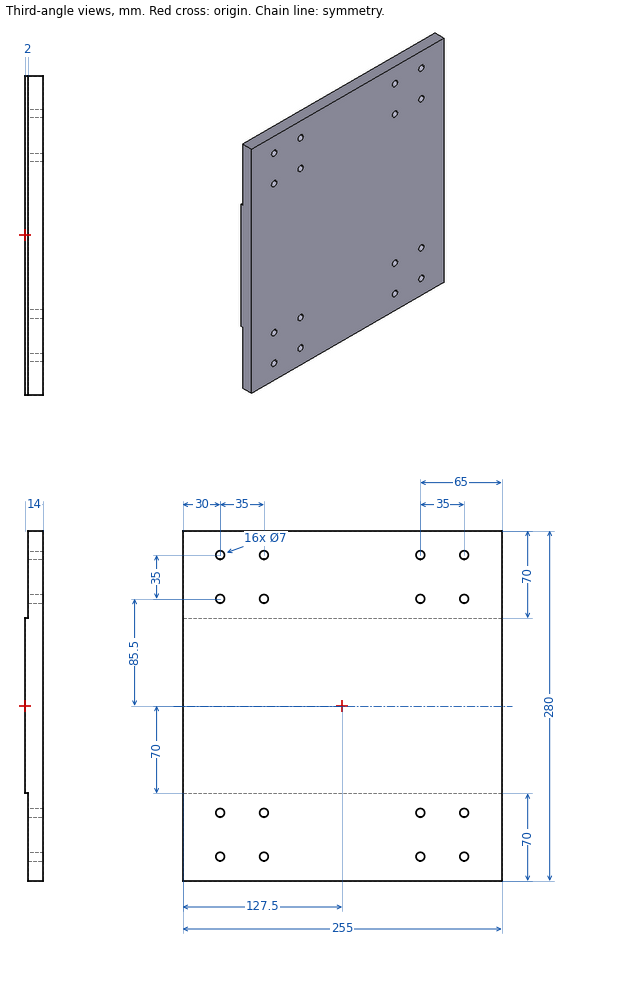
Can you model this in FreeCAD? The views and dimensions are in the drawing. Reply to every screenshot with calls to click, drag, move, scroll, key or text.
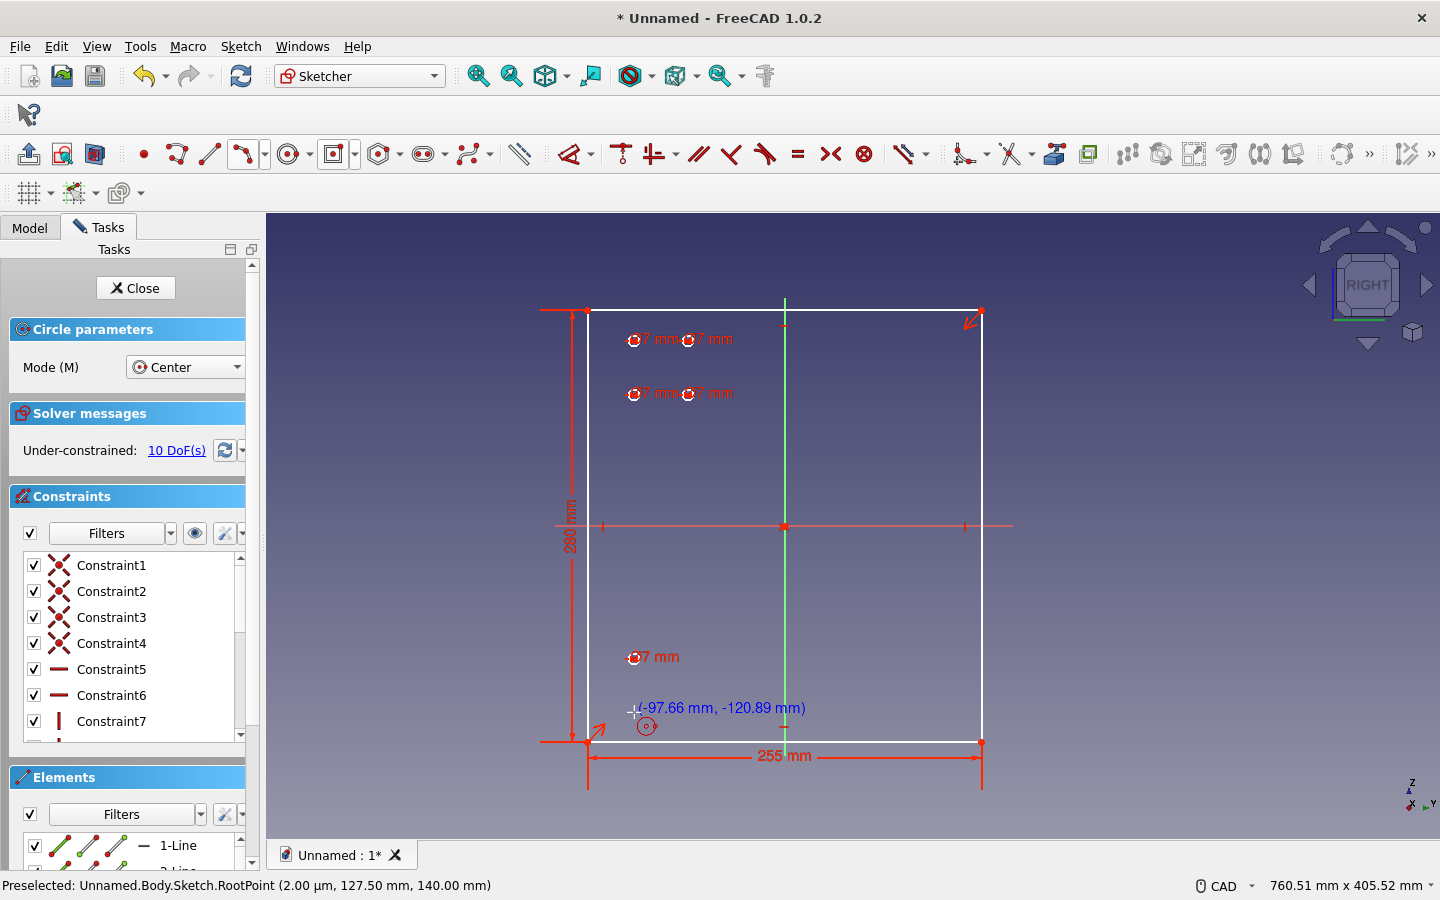
click(634, 712)
move(638, 709)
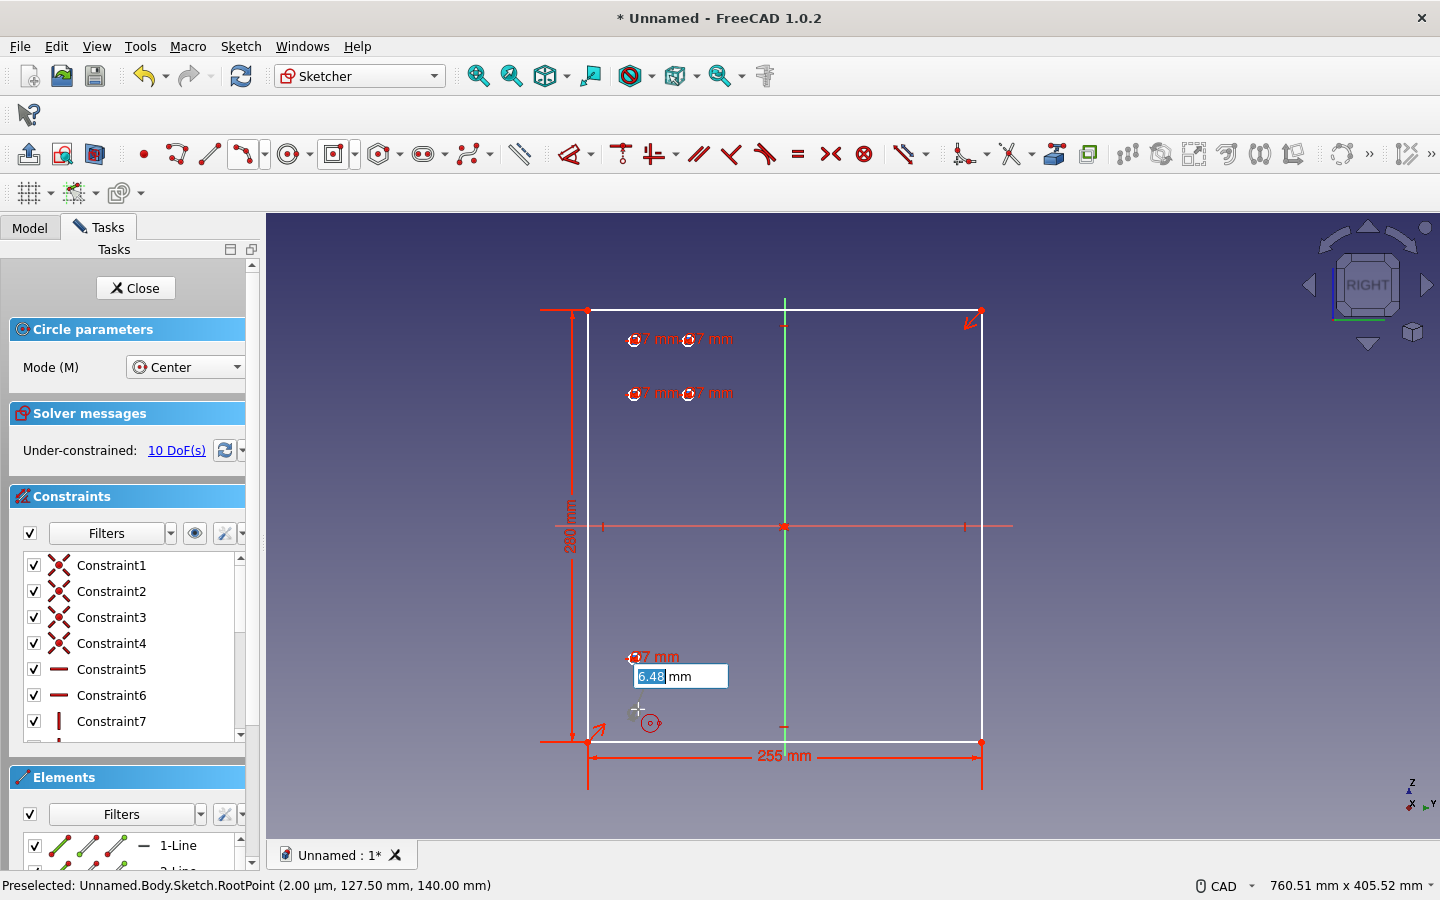
text(7)
key(Return)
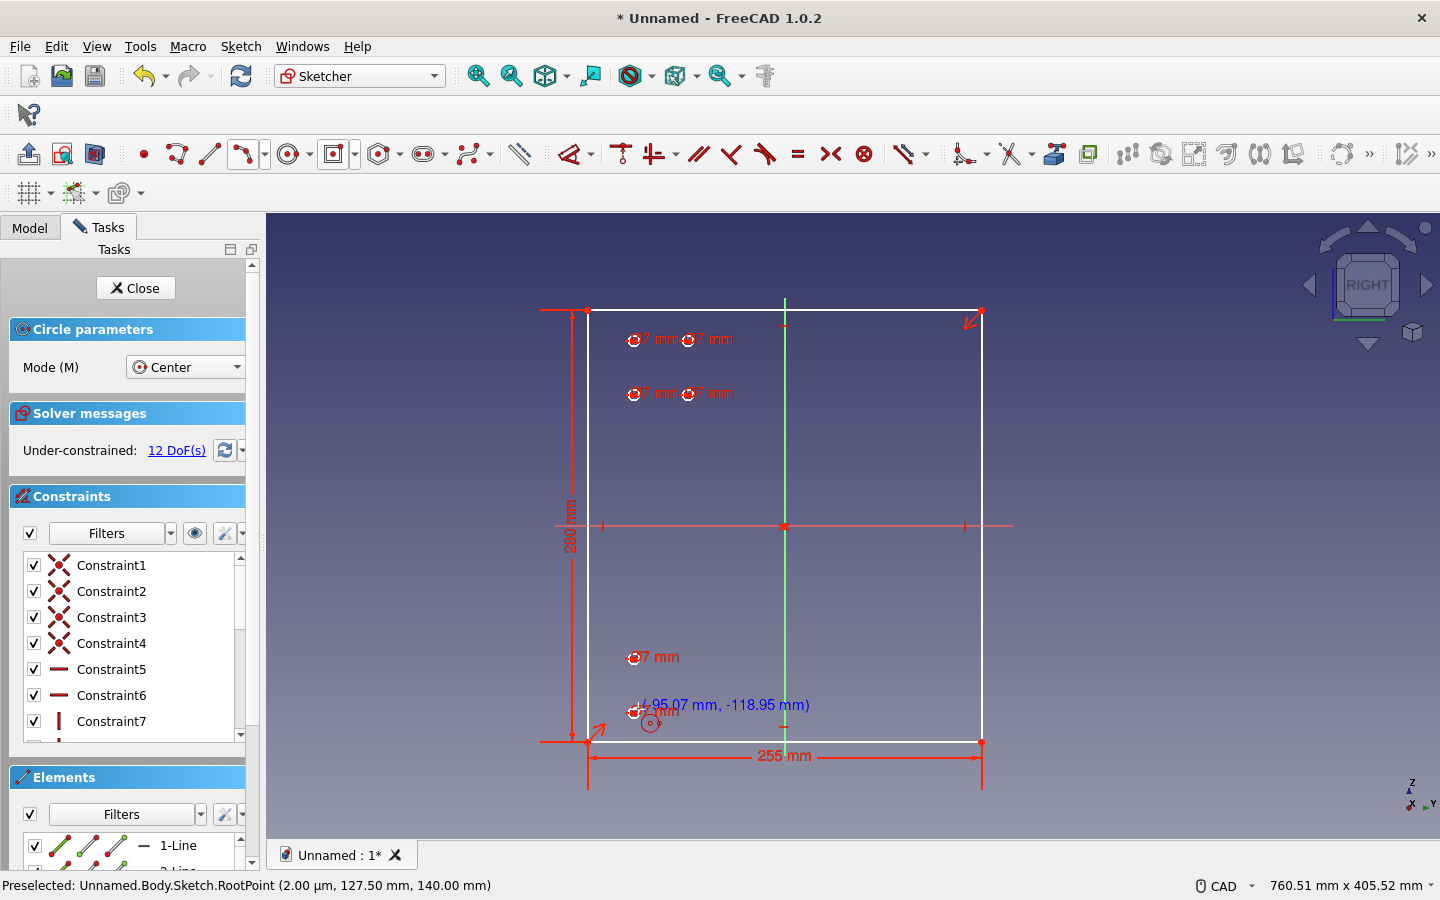
scroll(688, 658, up, 8)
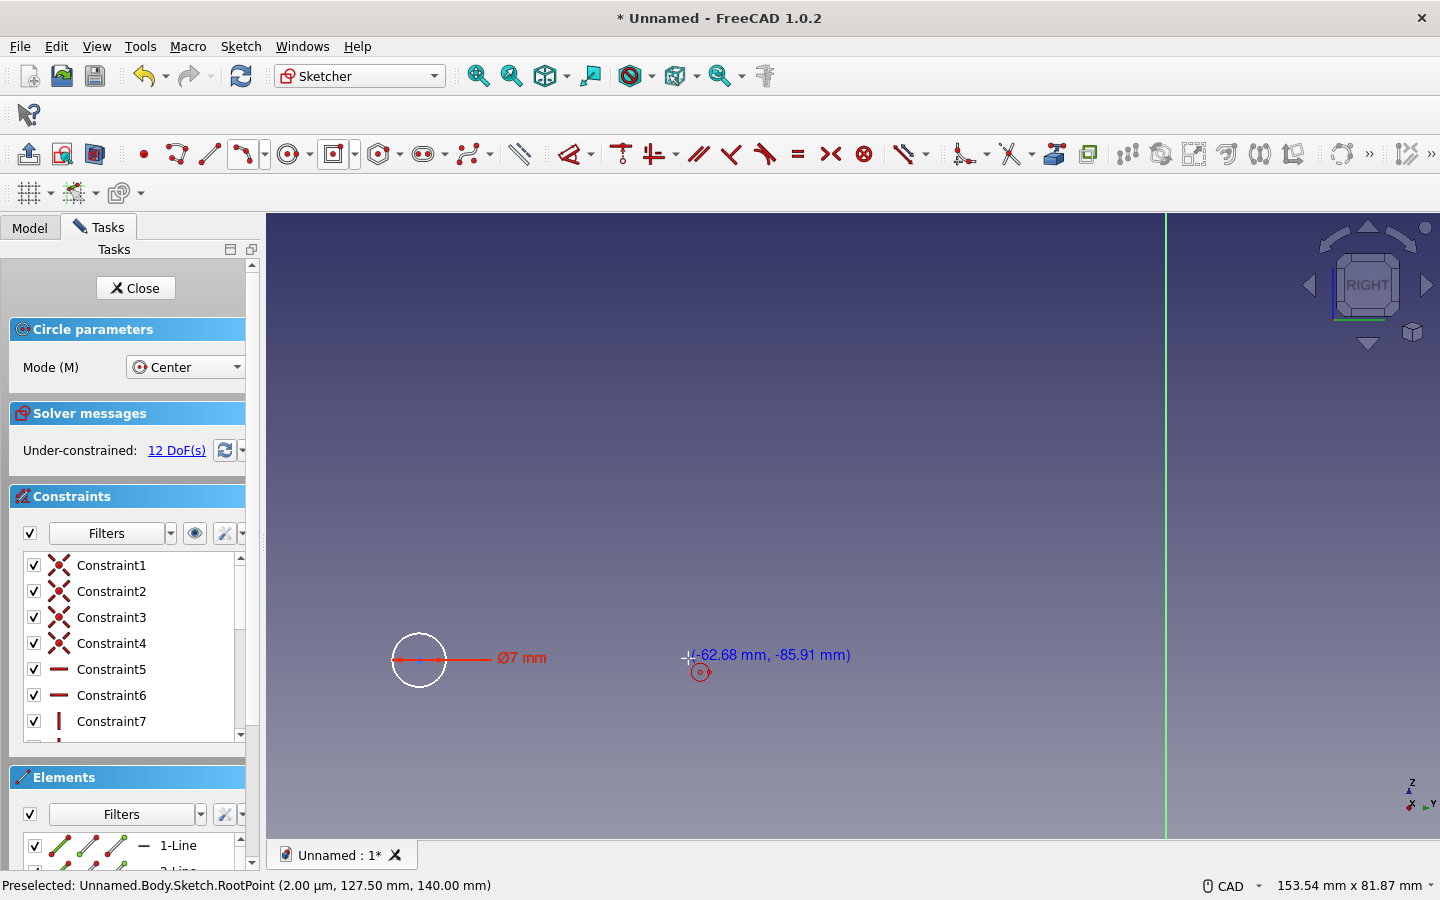
scroll(688, 658, down, 8)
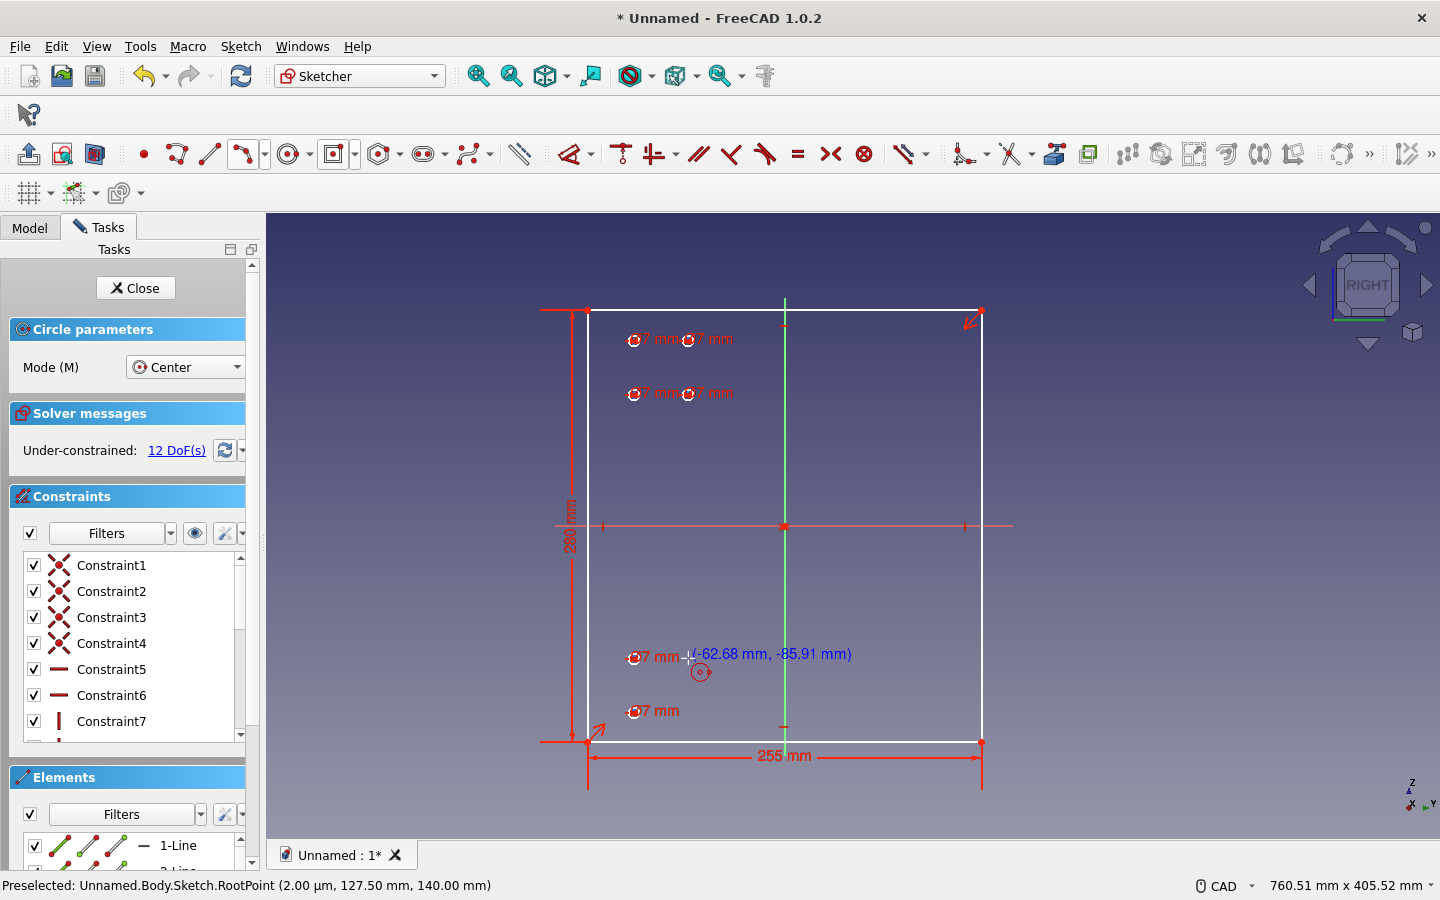
click(688, 658)
move(692, 655)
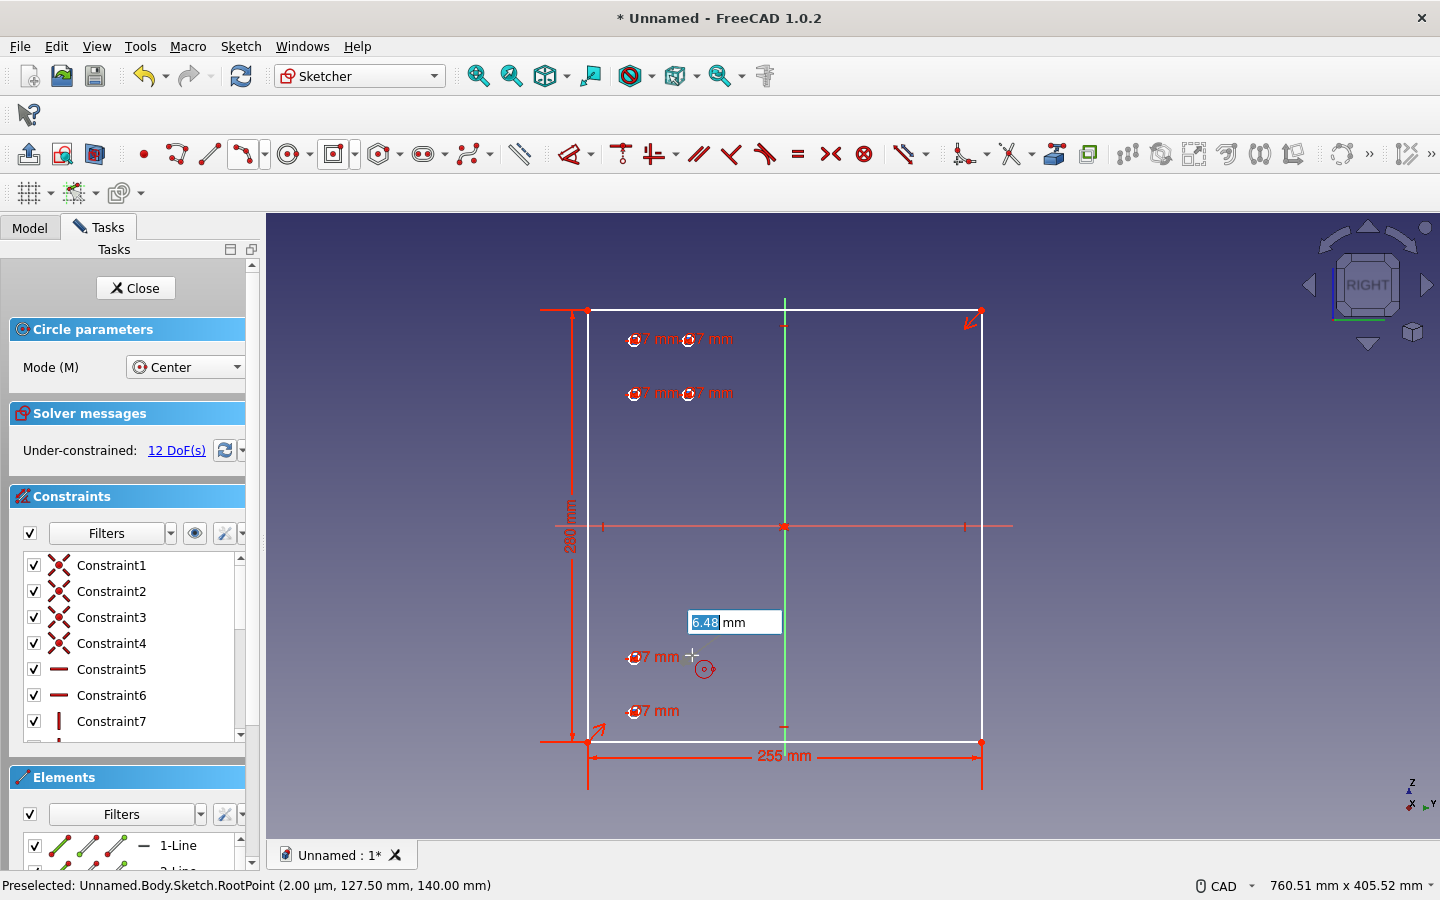
text(7)
key(Return)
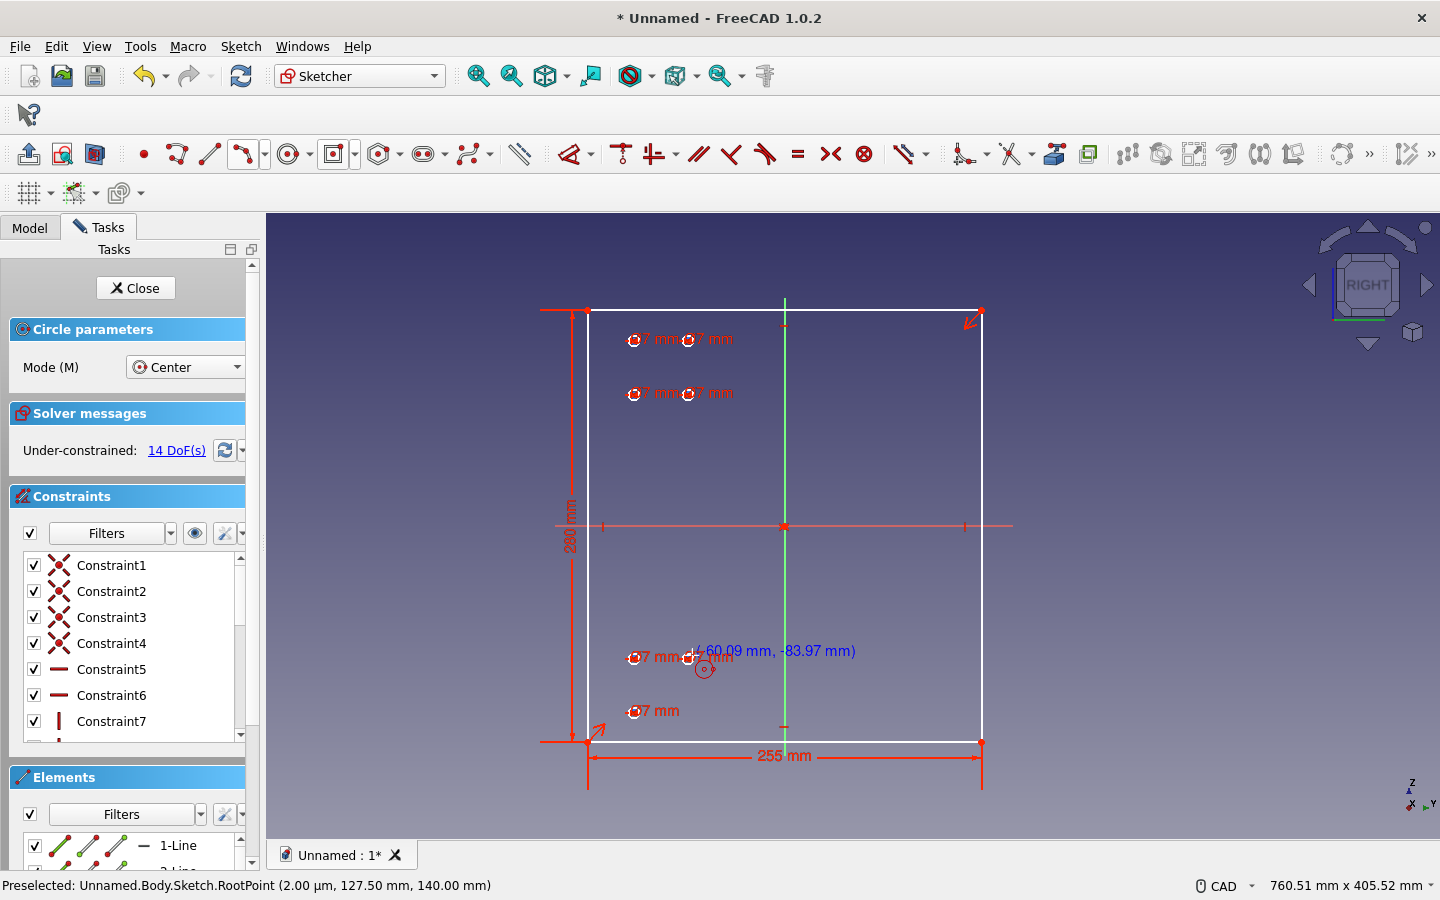
scroll(688, 712, up, 8)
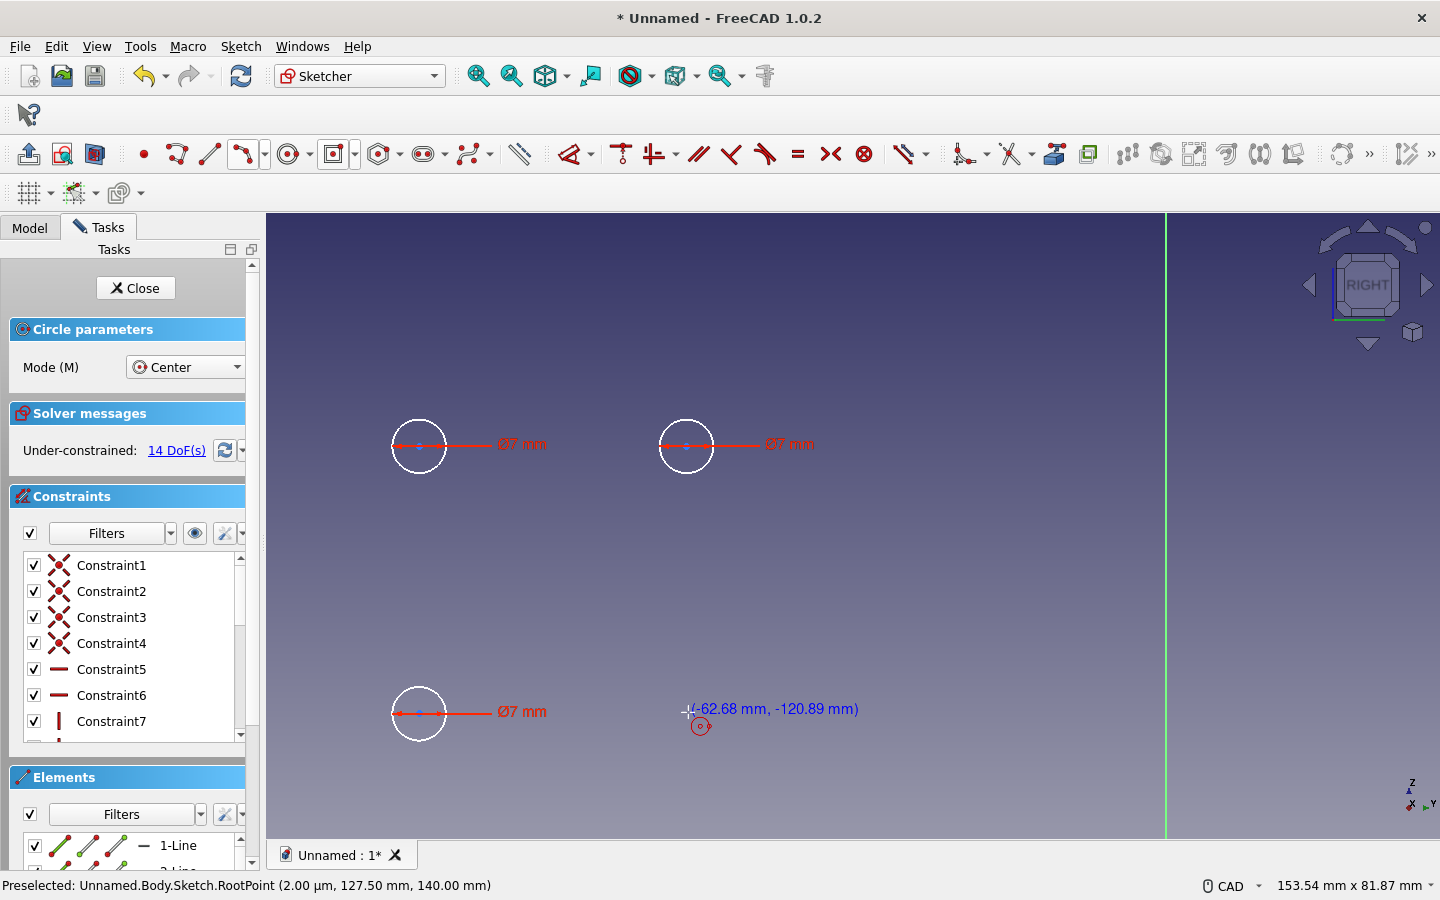
scroll(688, 712, down, 8)